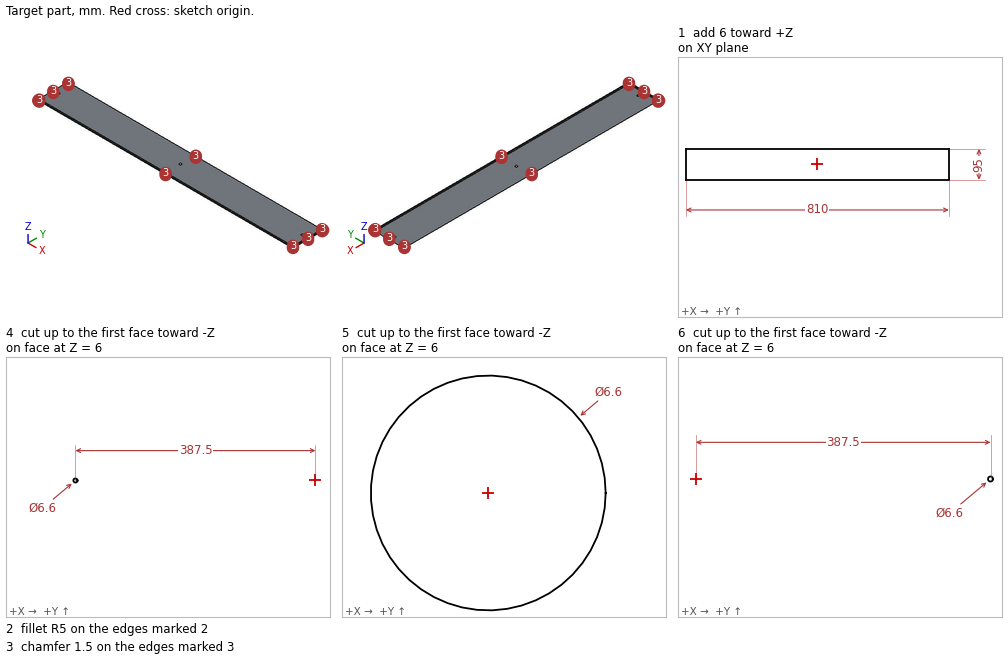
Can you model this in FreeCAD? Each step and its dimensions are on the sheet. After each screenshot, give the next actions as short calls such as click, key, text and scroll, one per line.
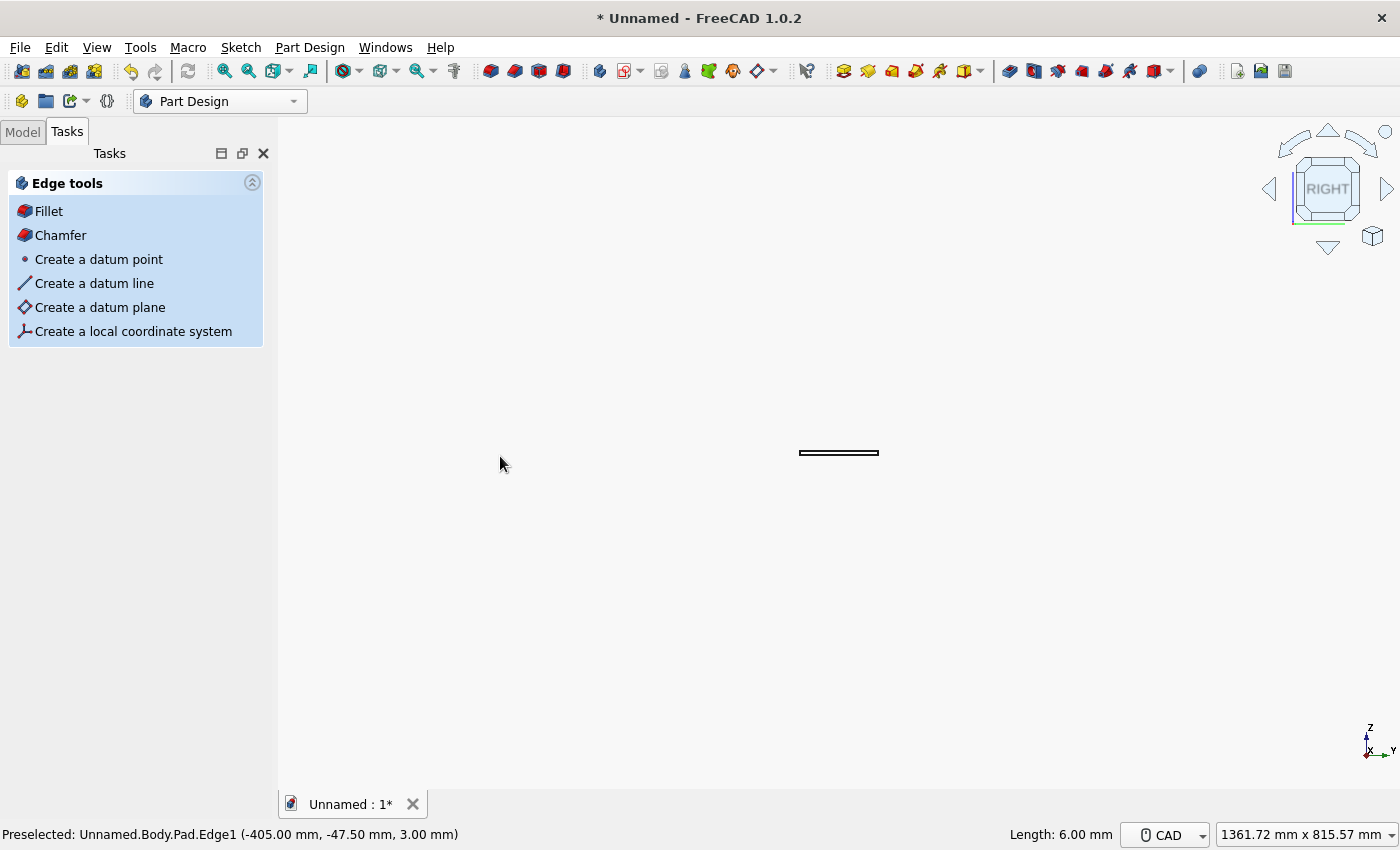
scroll(878, 452, up, 11)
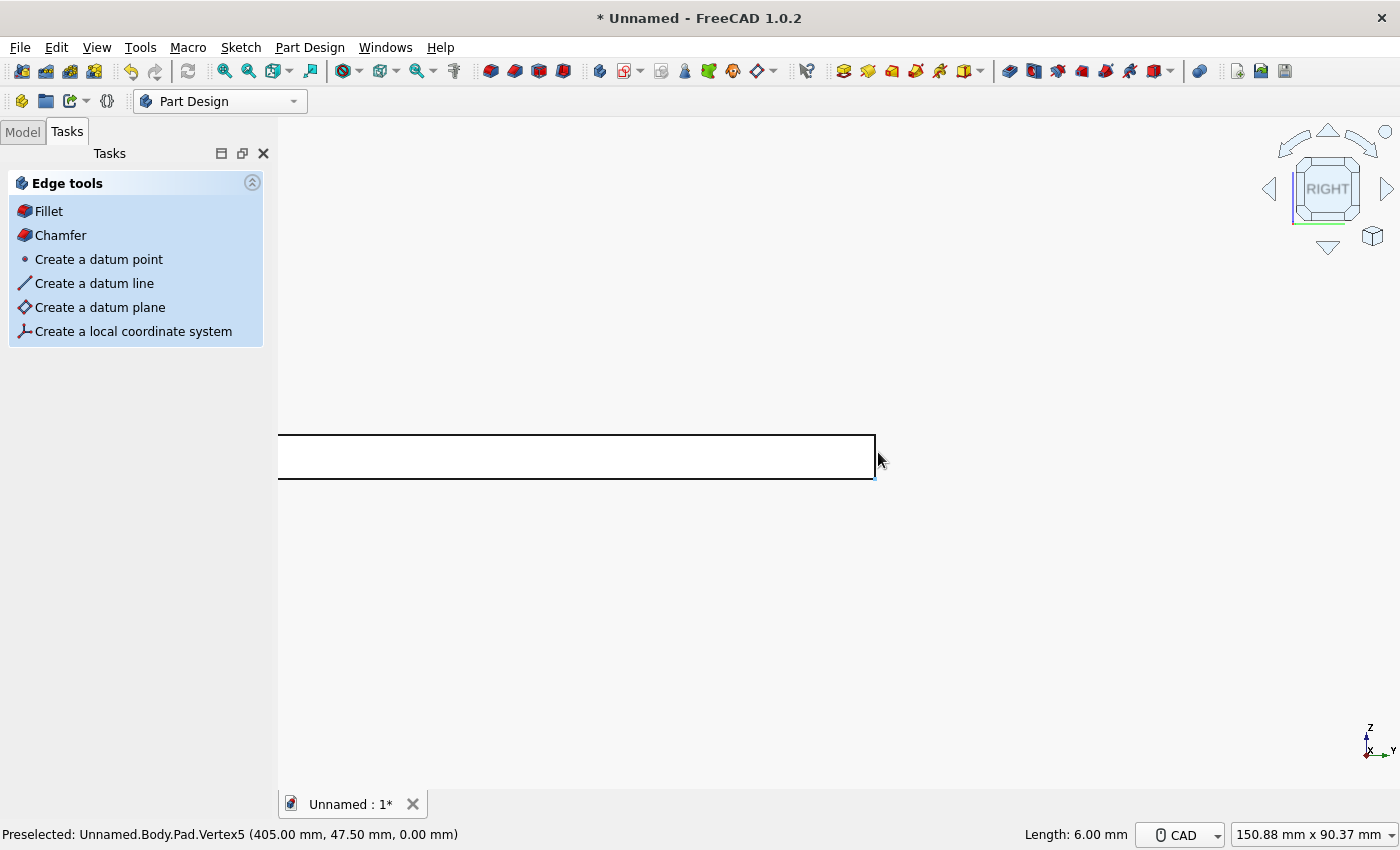
click(875, 456, ctrl)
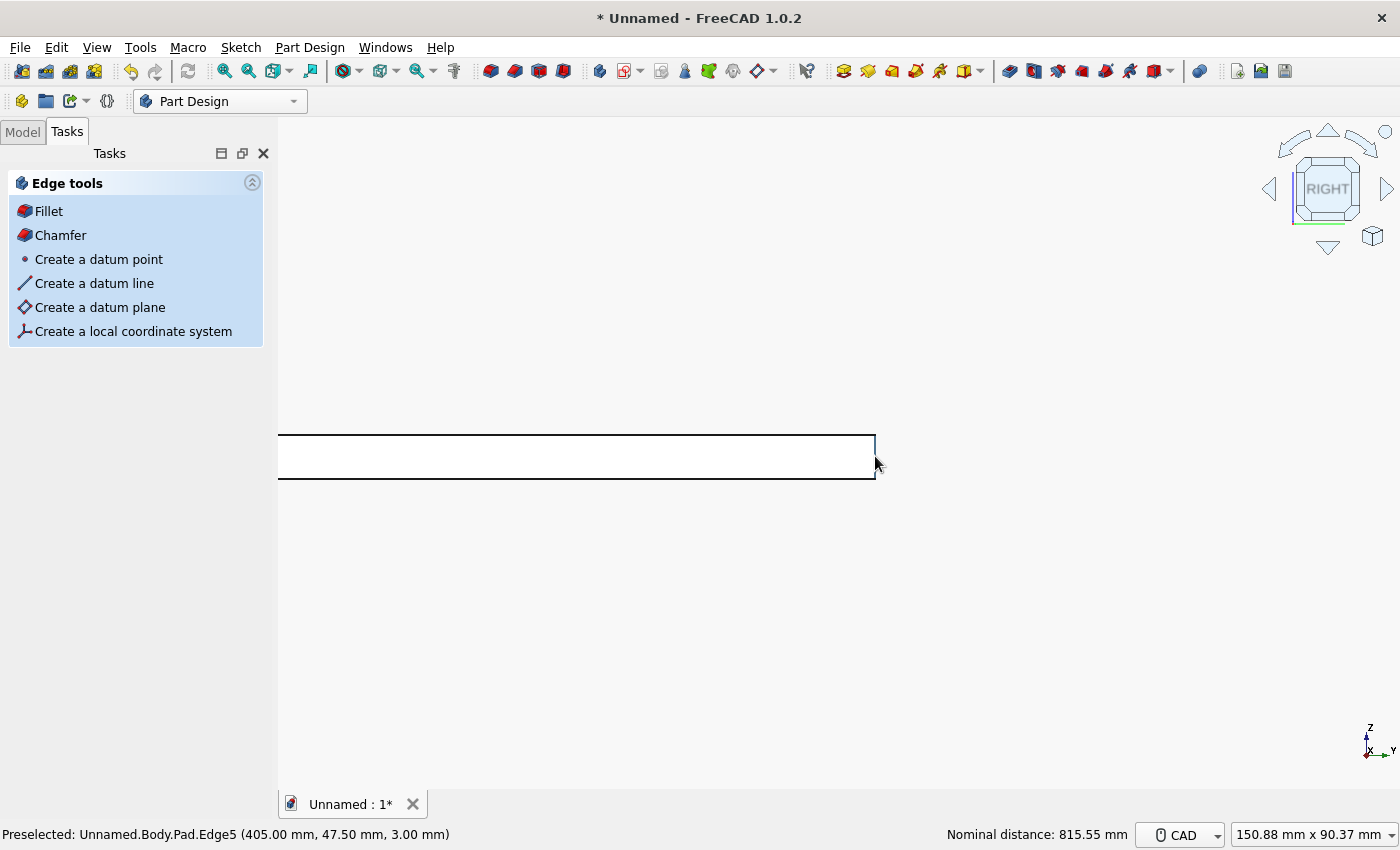
key(v)
key(f)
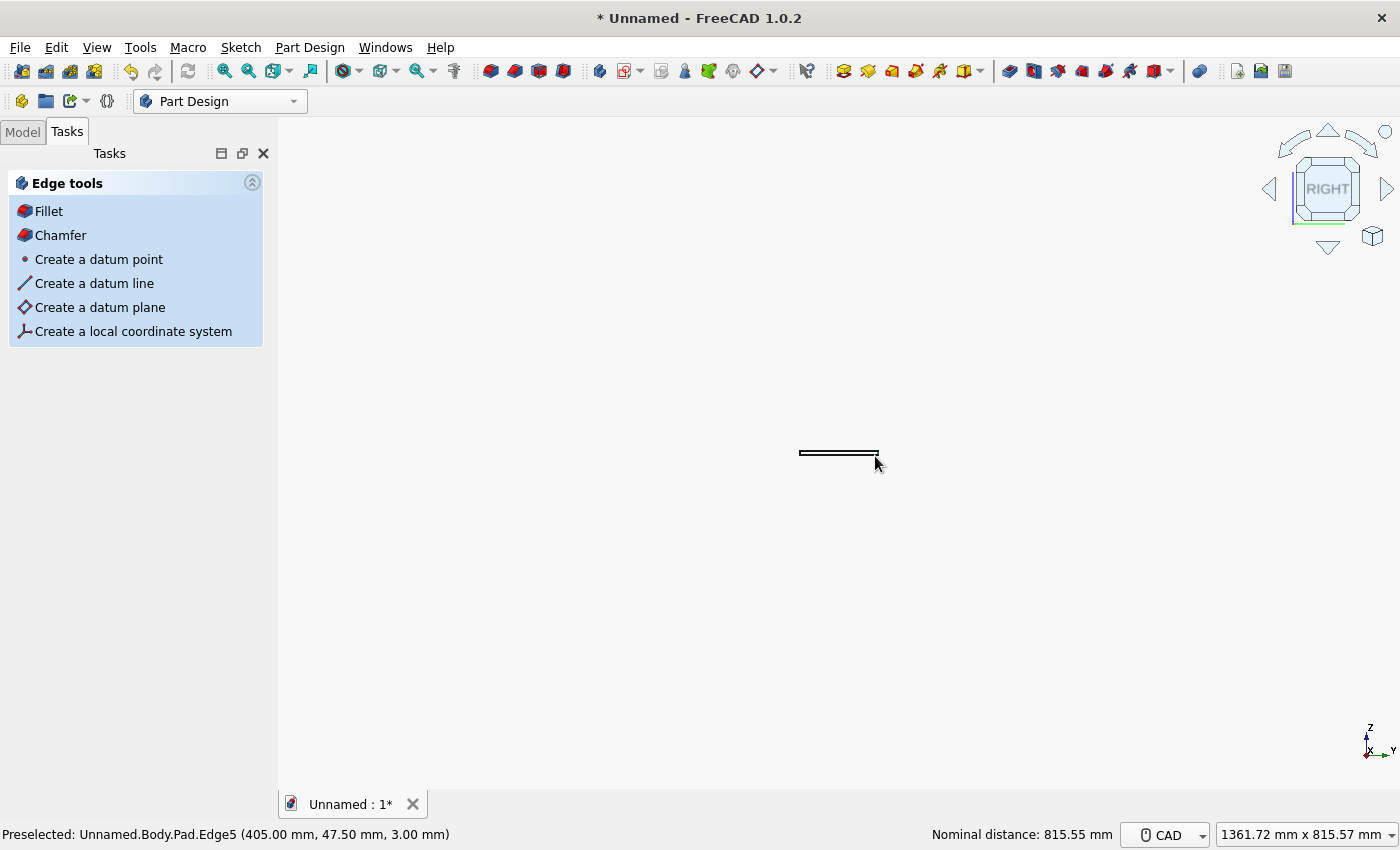
key(5)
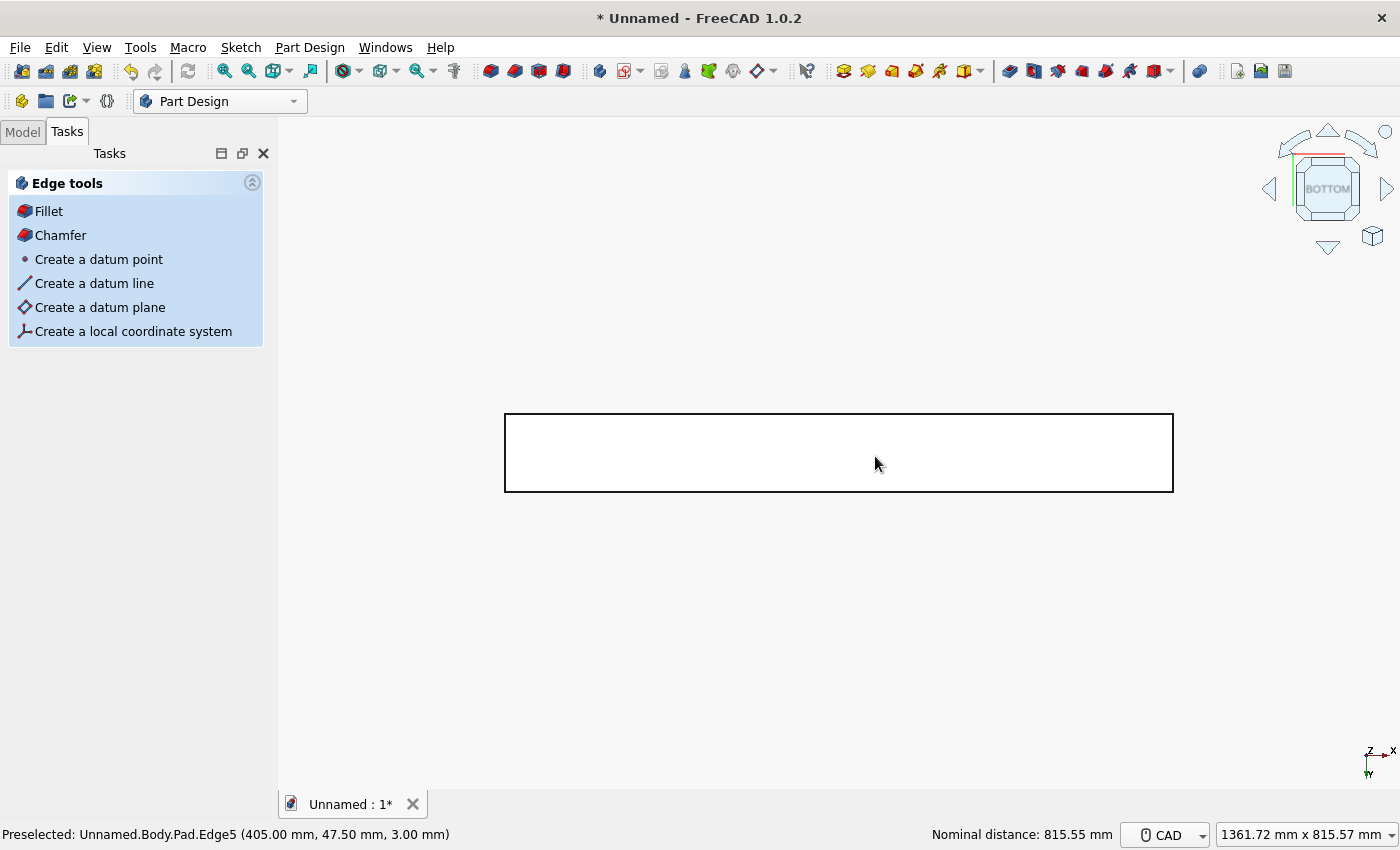
scroll(505, 491, up, 11)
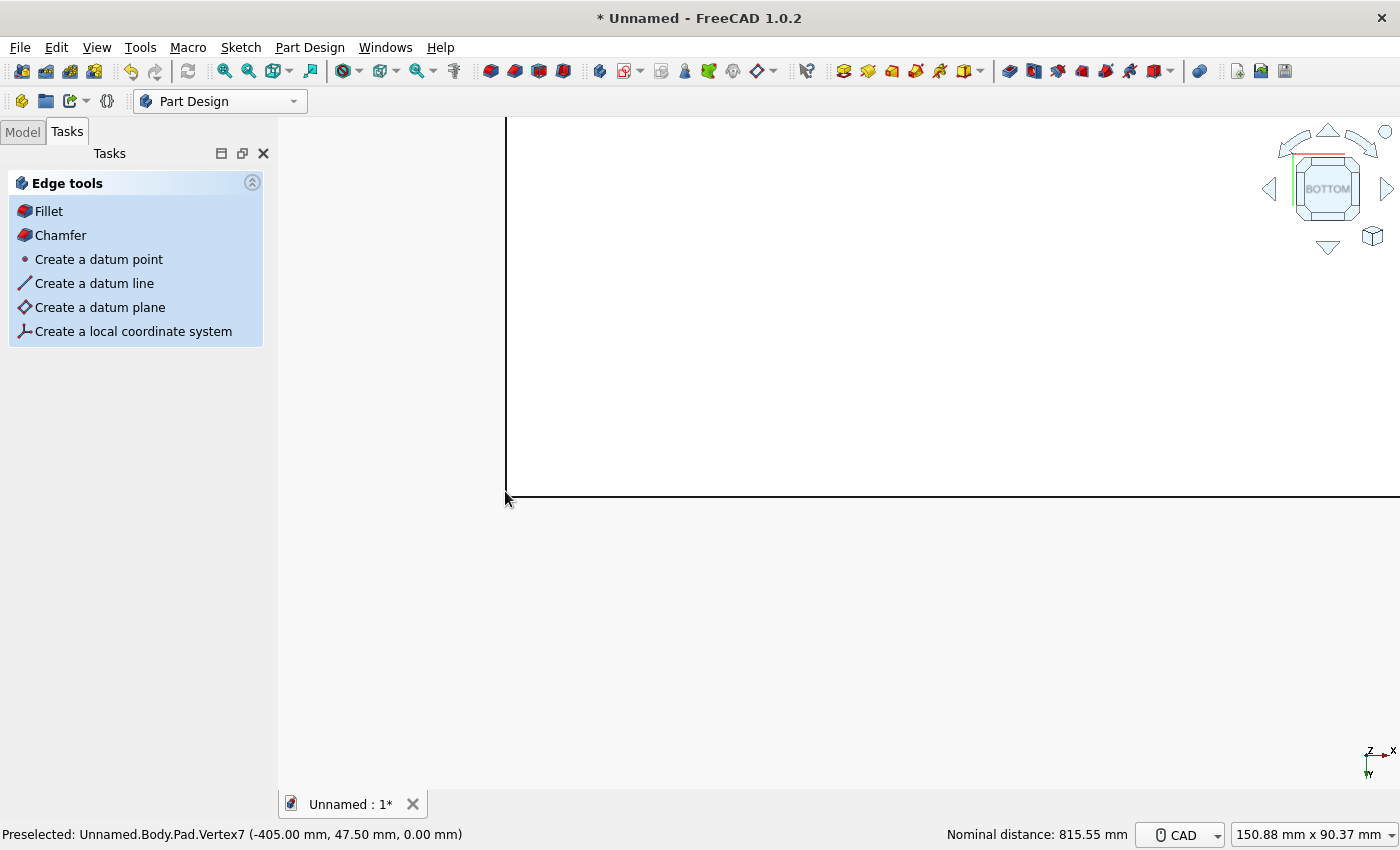
key(v)
key(f)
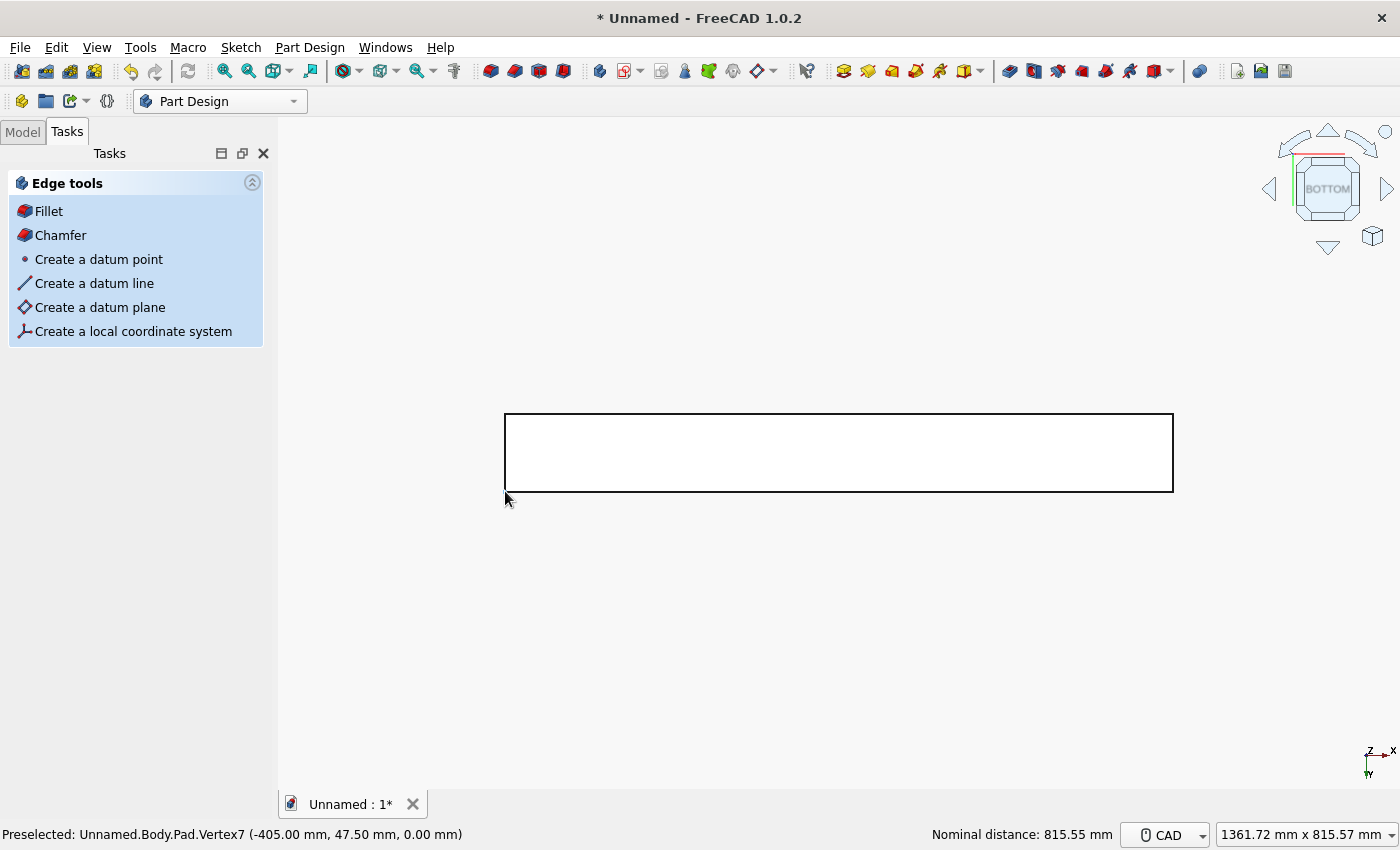
key(4)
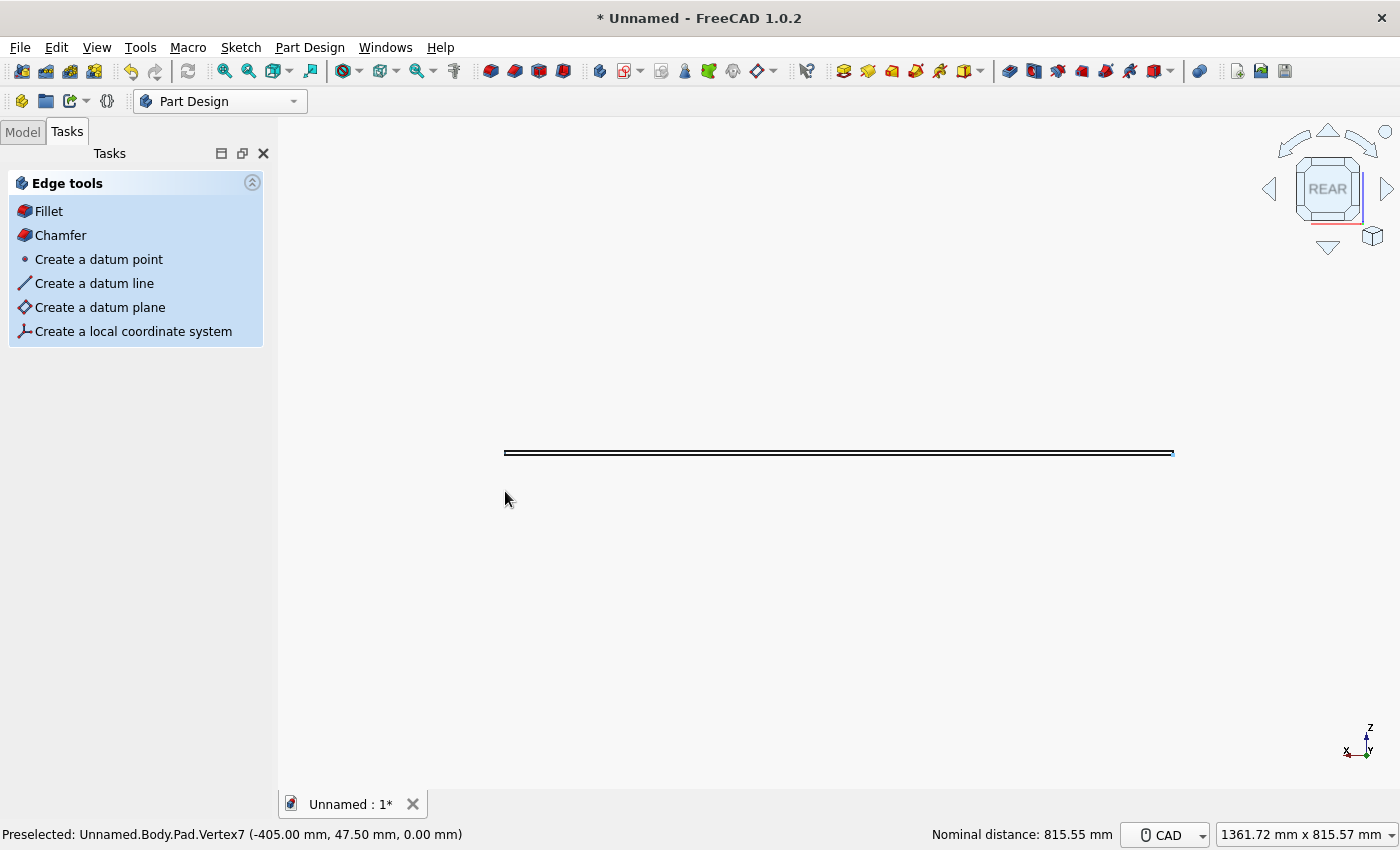
scroll(1173, 452, up, 11)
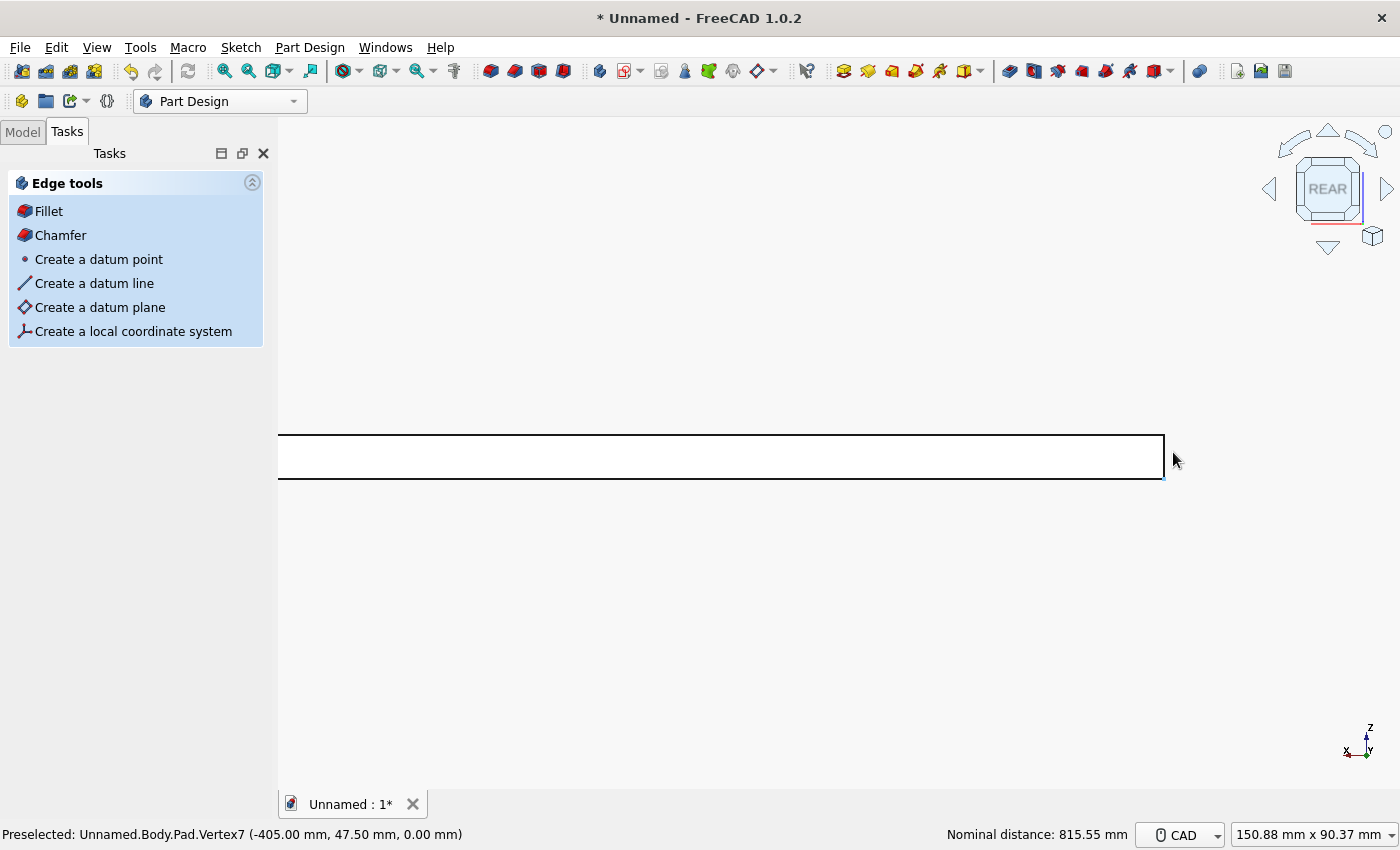
click(1164, 456, ctrl)